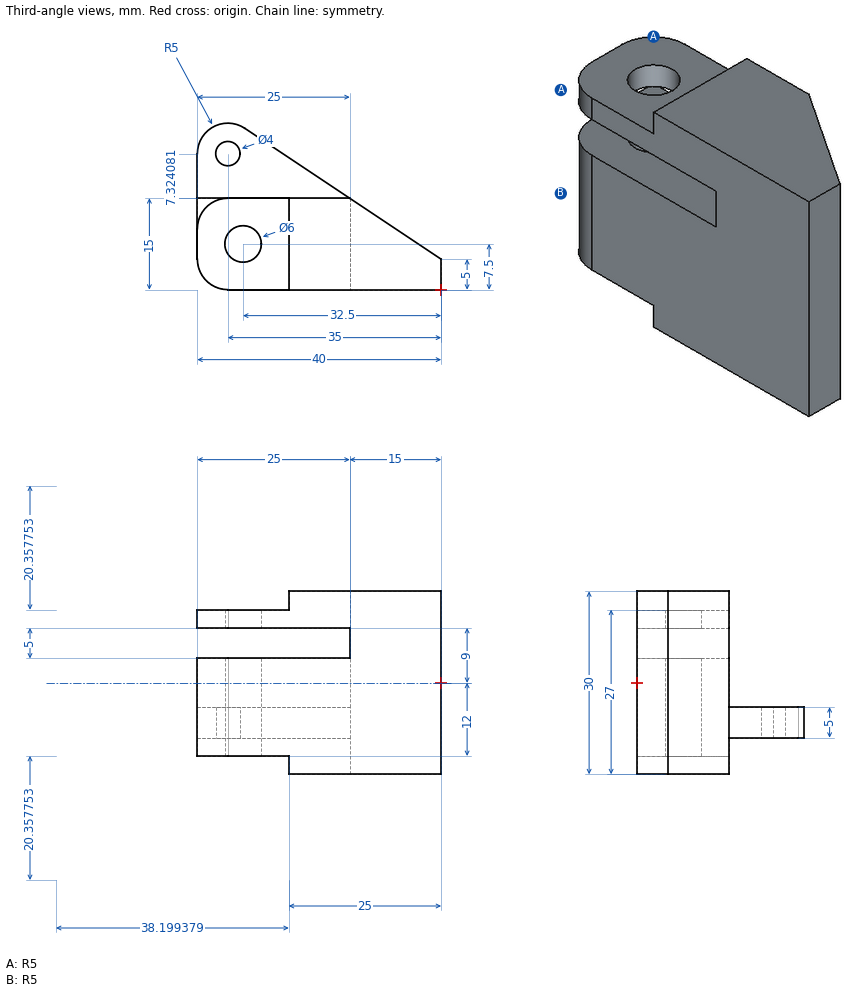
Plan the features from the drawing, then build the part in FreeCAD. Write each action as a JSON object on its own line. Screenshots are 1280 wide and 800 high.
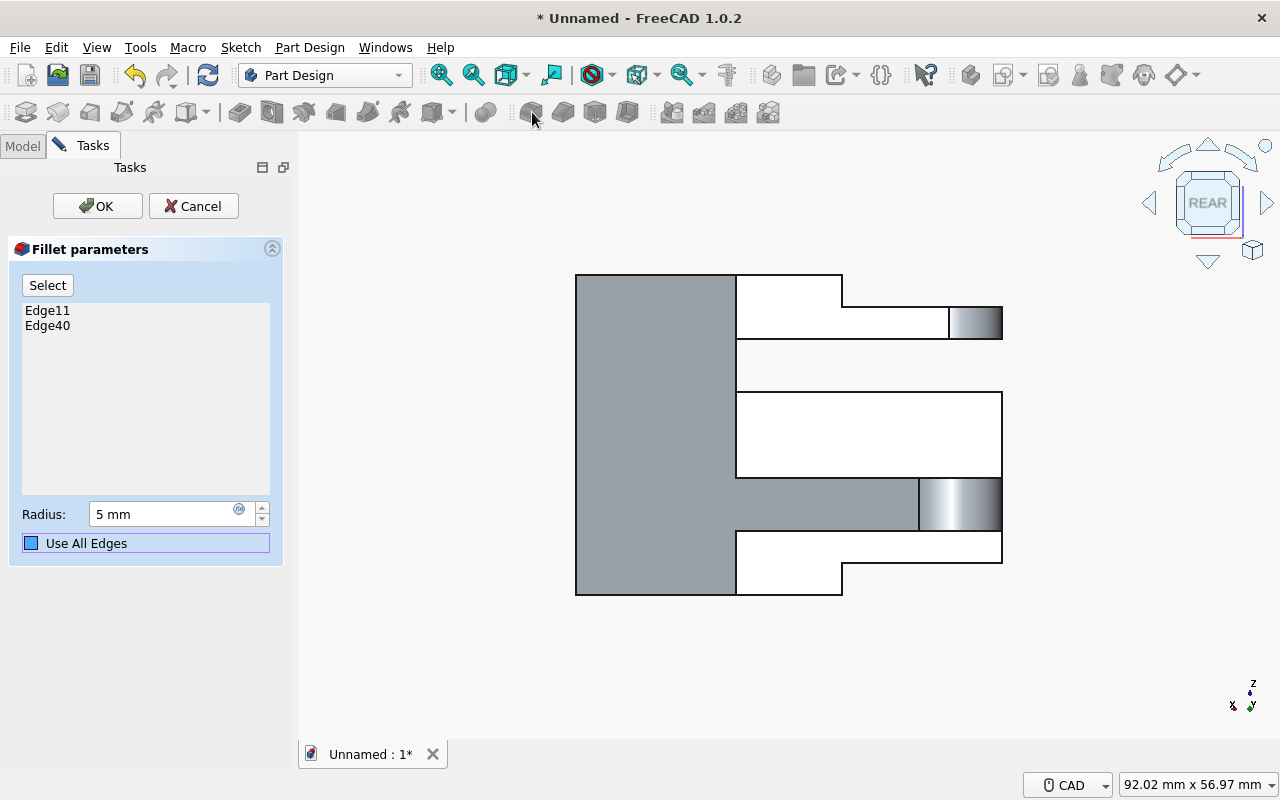
{"action": "left_click", "coordinate": [98, 206]}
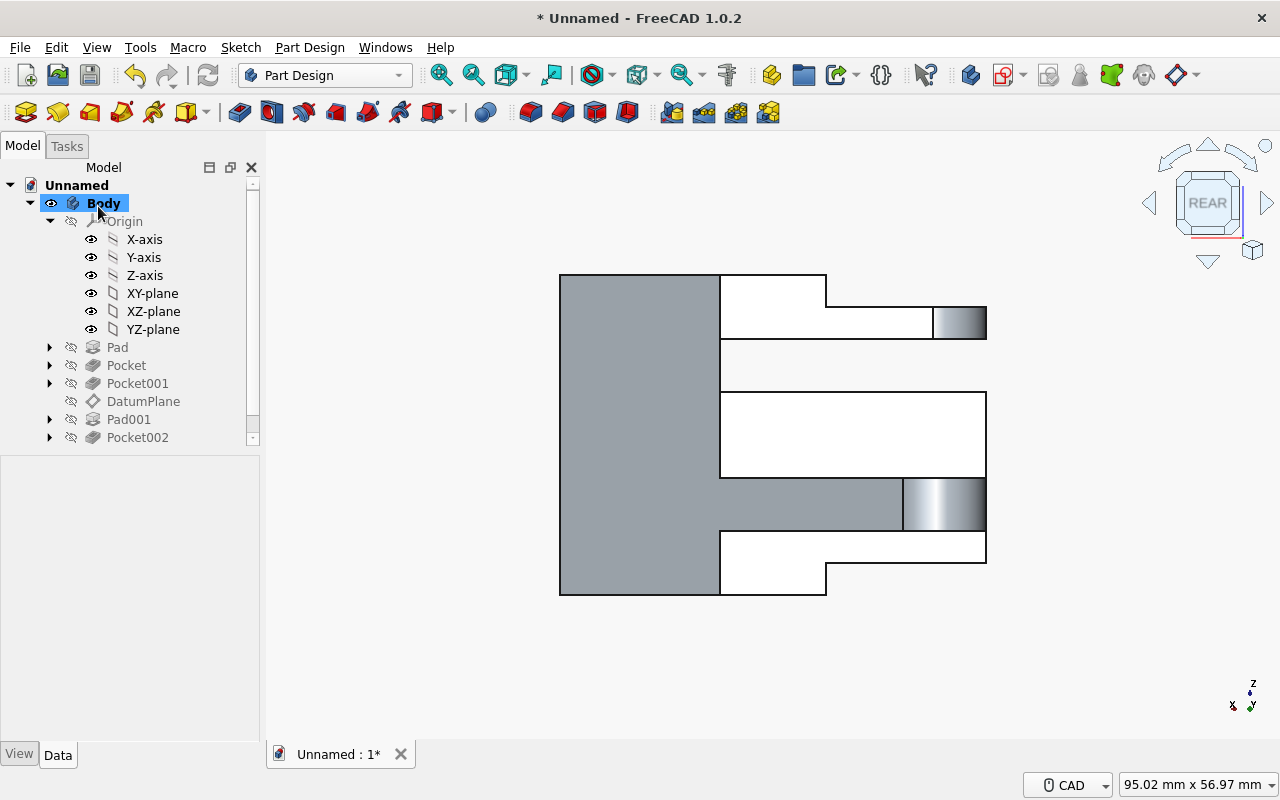
{"action": "key", "text": "0"}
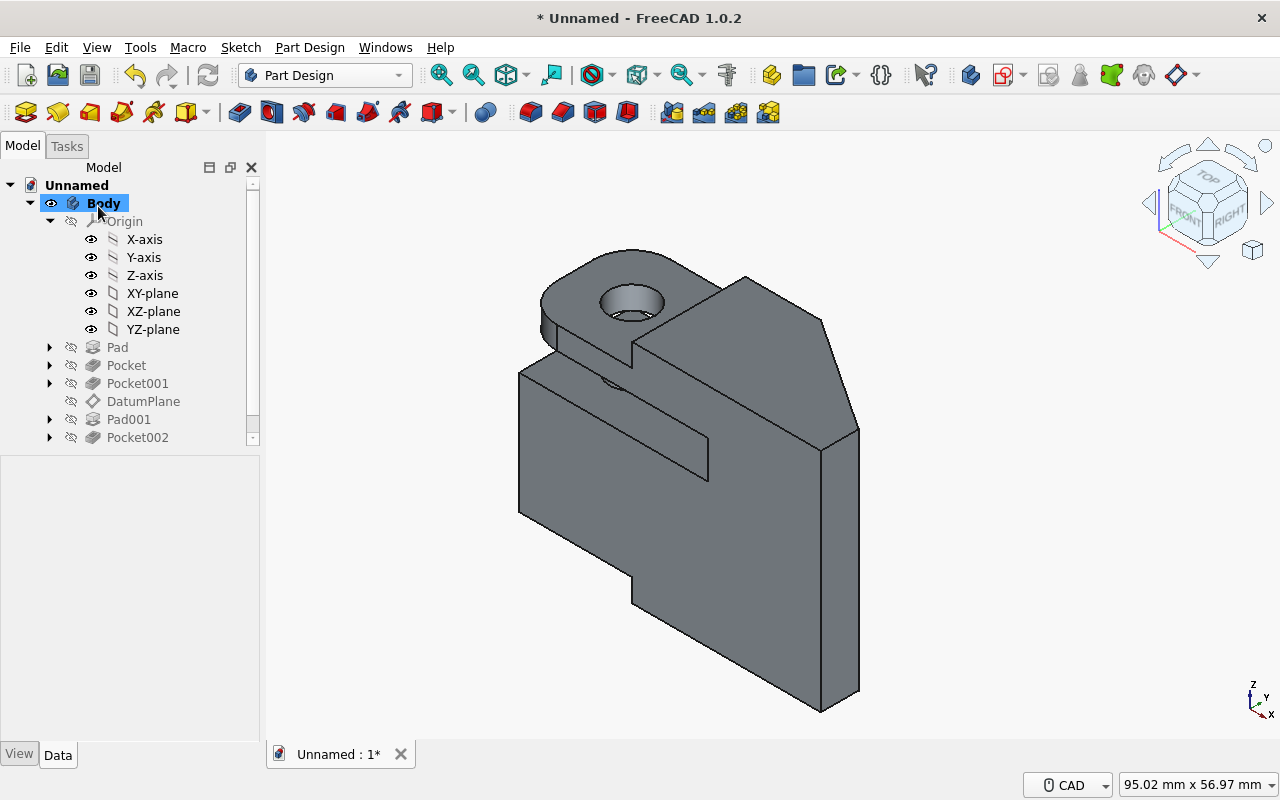
{"action": "key", "text": "2"}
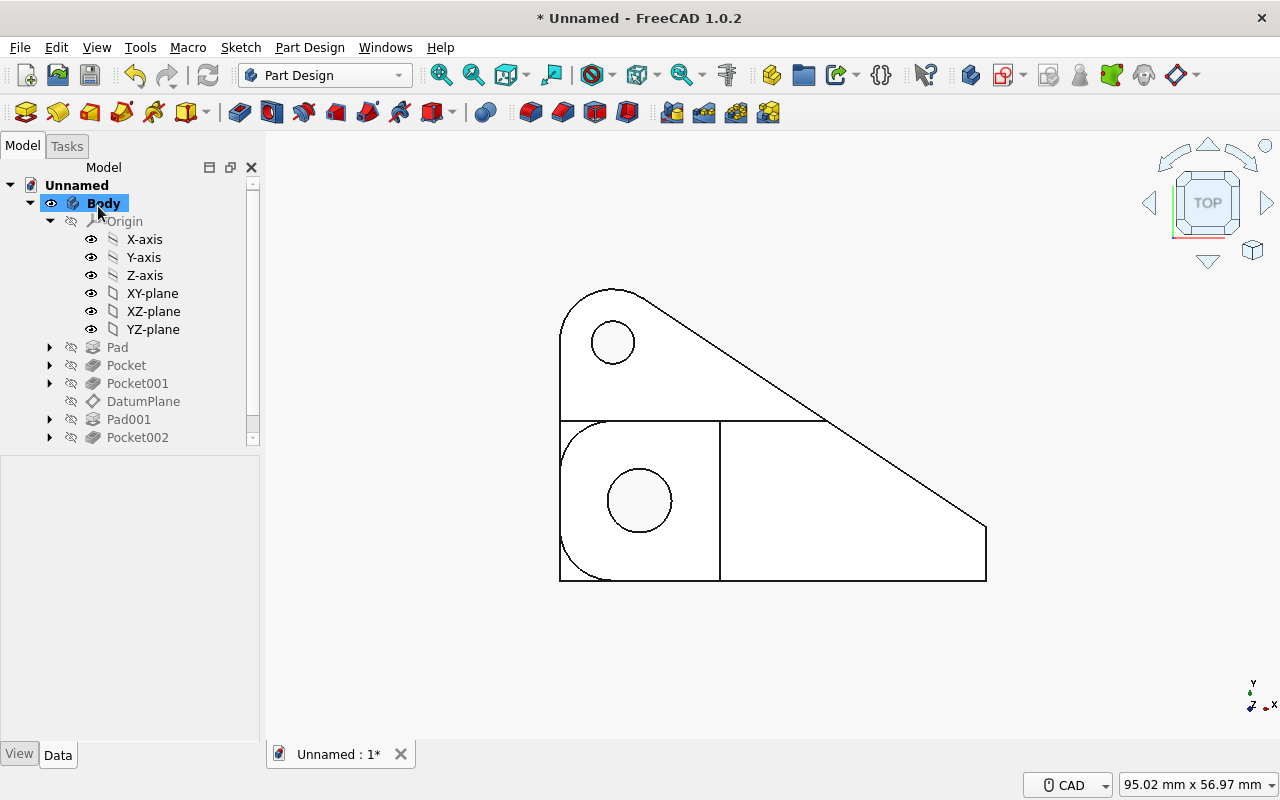
{"action": "key", "text": "1"}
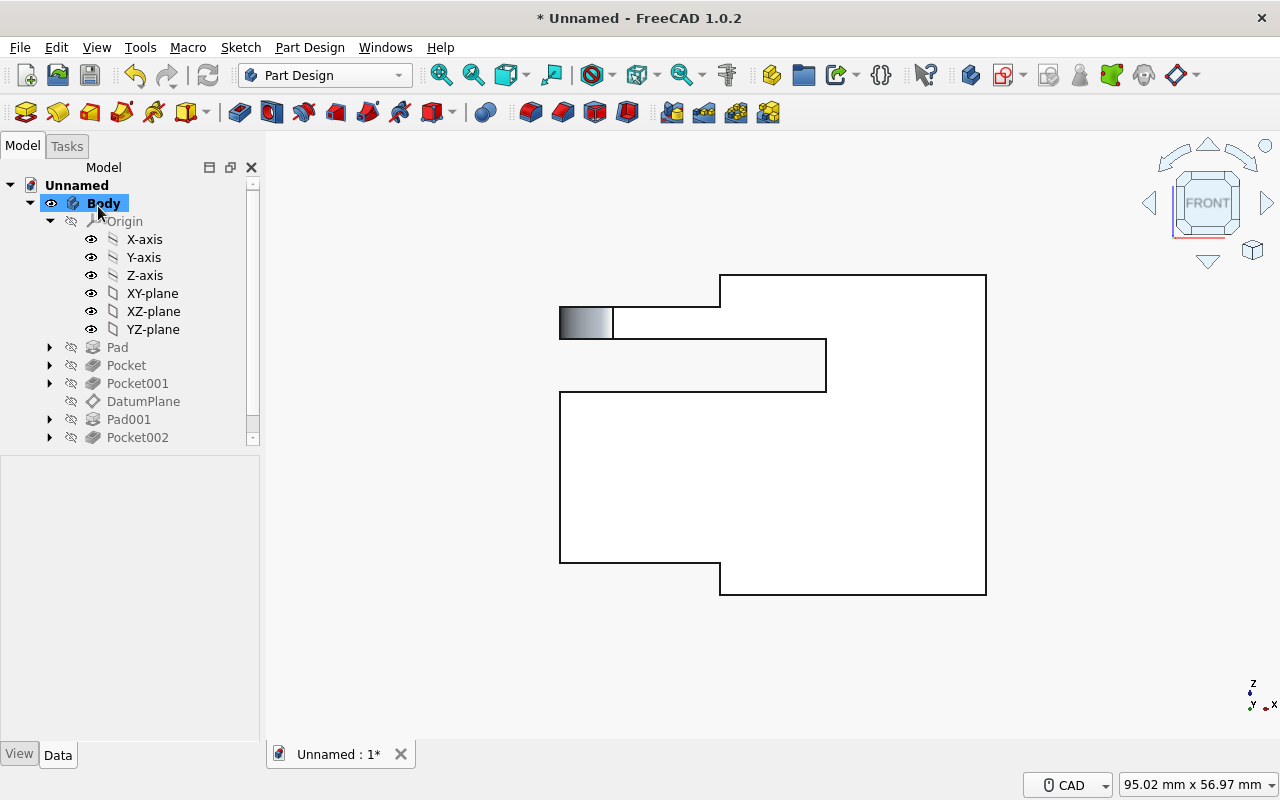
{"action": "left_click", "coordinate": [560, 477]}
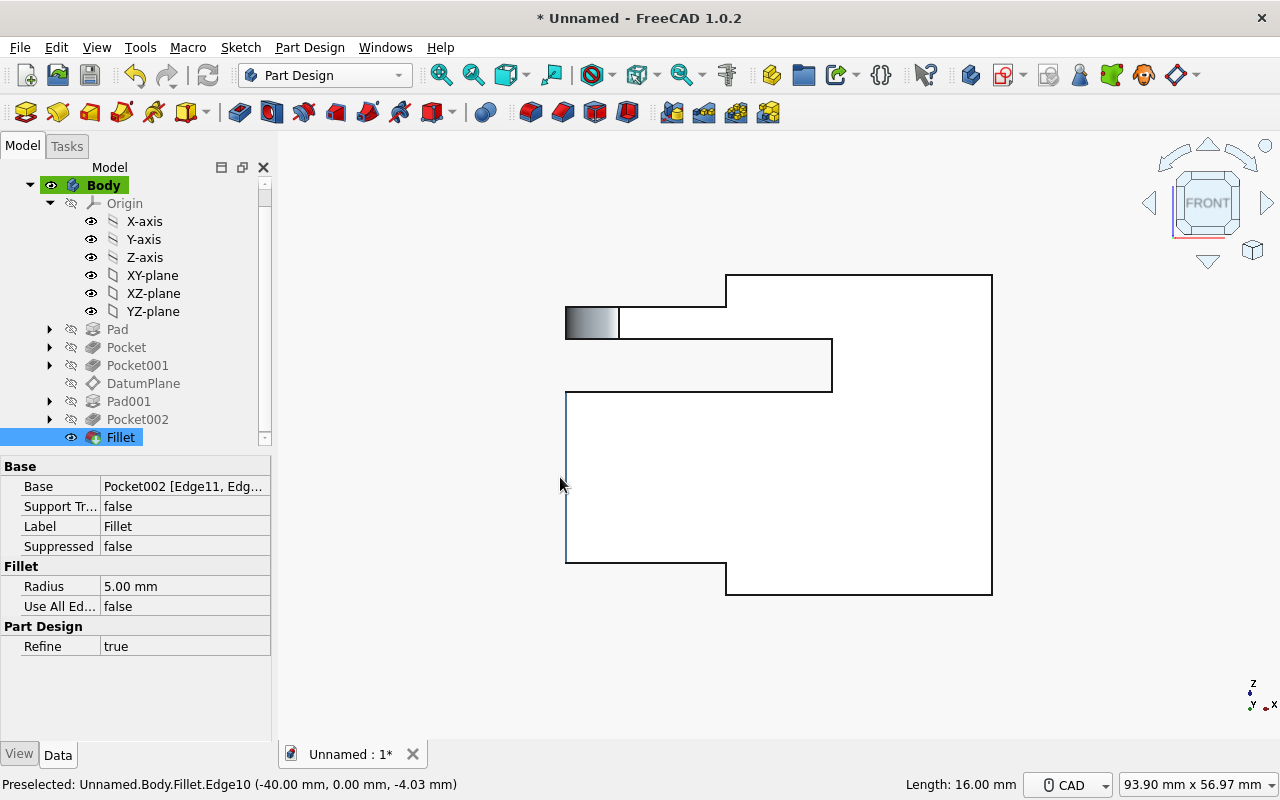
{"action": "left_click", "coordinate": [532, 112]}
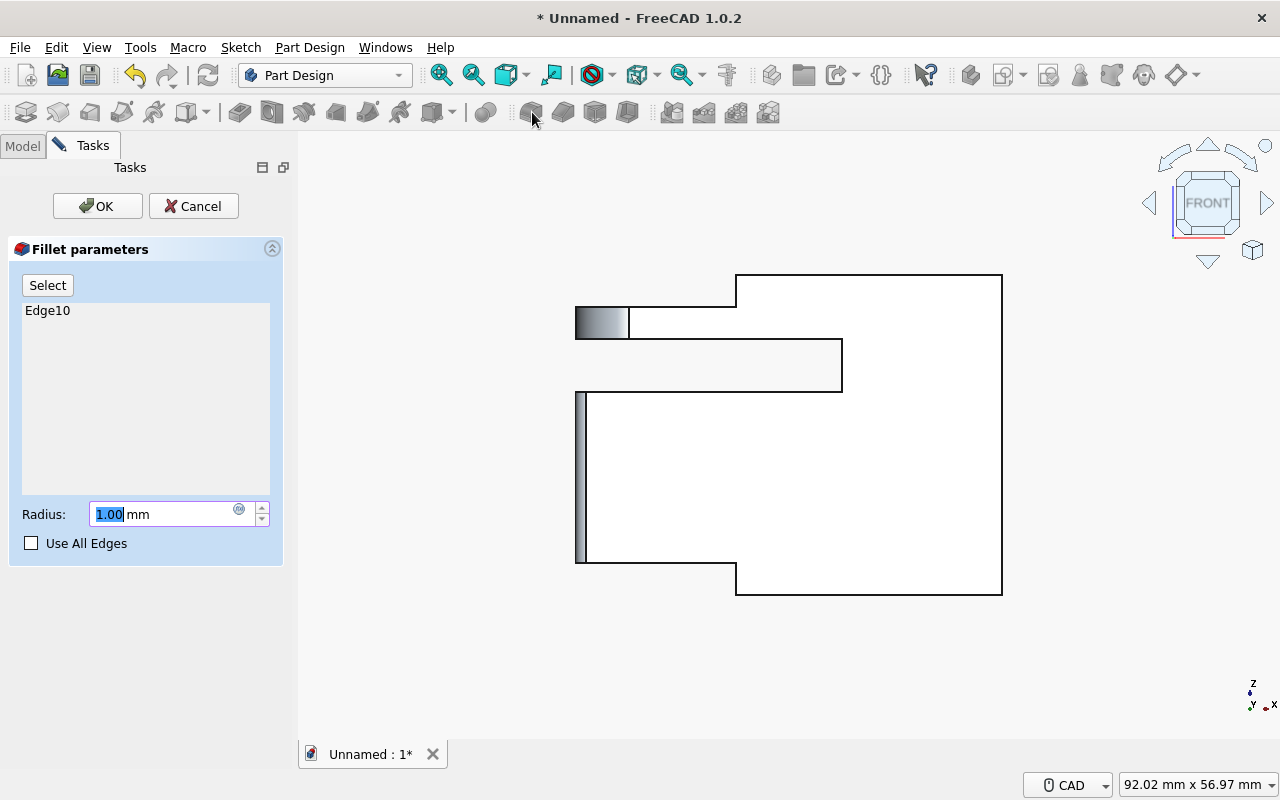
{"action": "type", "text": "5"}
{"action": "key", "text": "Tab"}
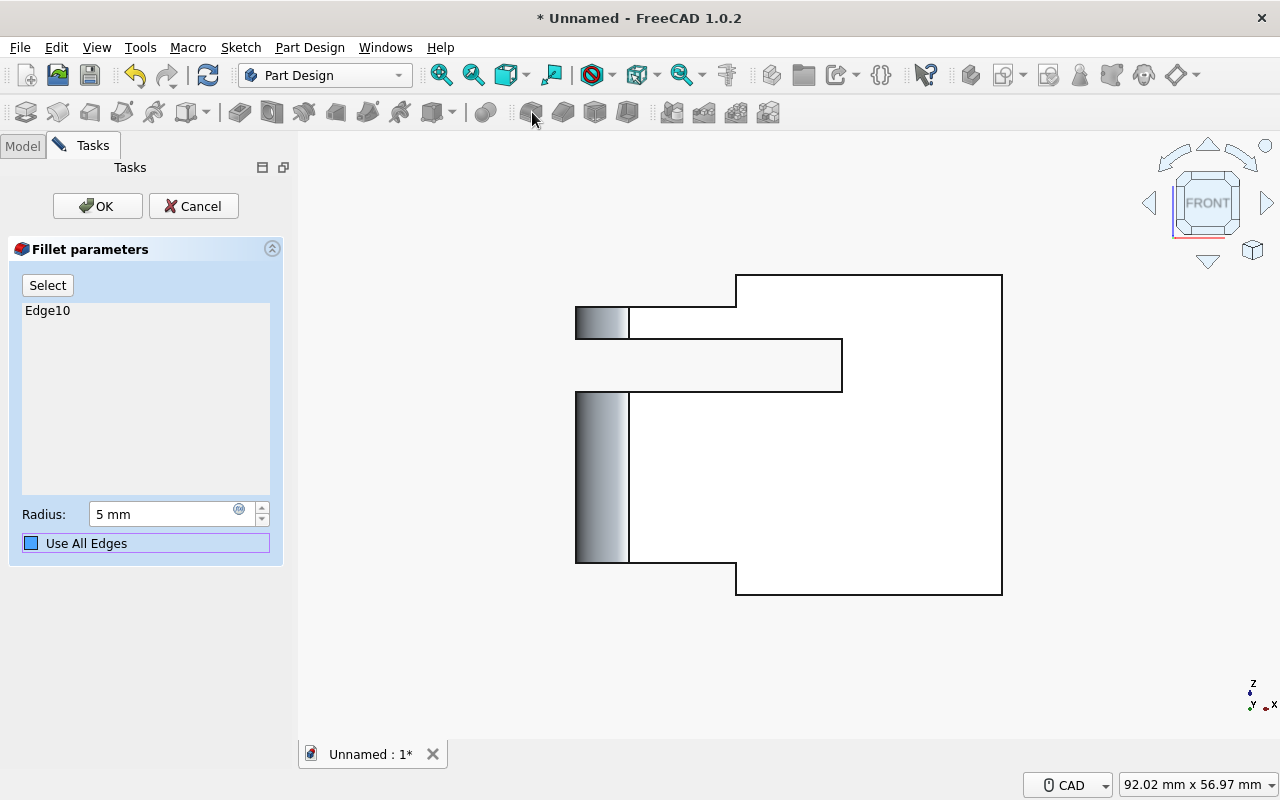
{"action": "left_click", "coordinate": [98, 206]}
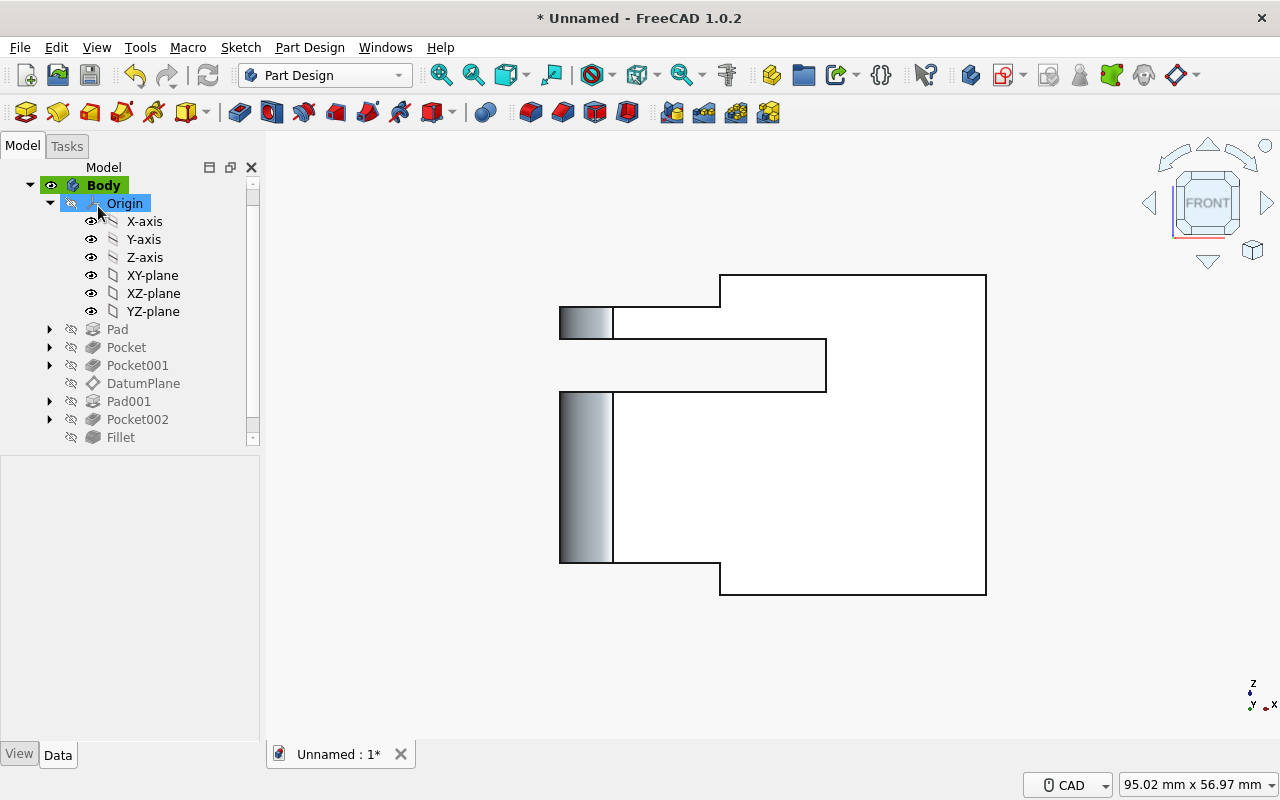
{"action": "key", "text": "0"}